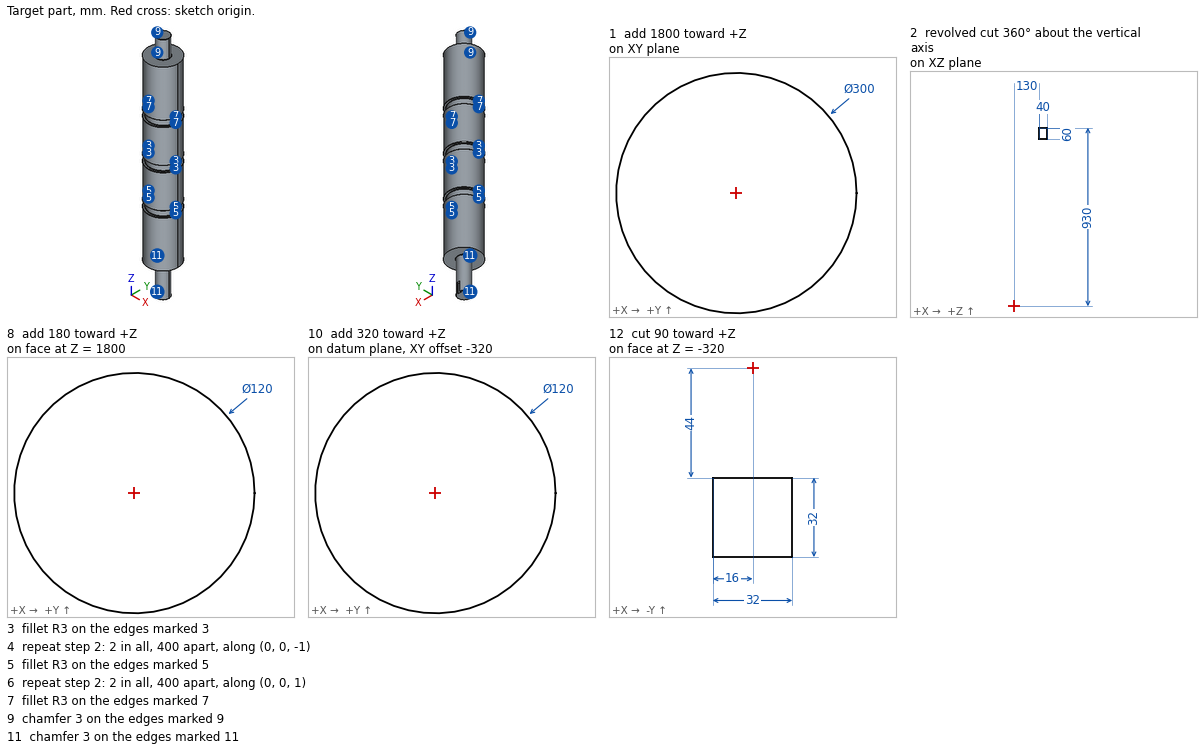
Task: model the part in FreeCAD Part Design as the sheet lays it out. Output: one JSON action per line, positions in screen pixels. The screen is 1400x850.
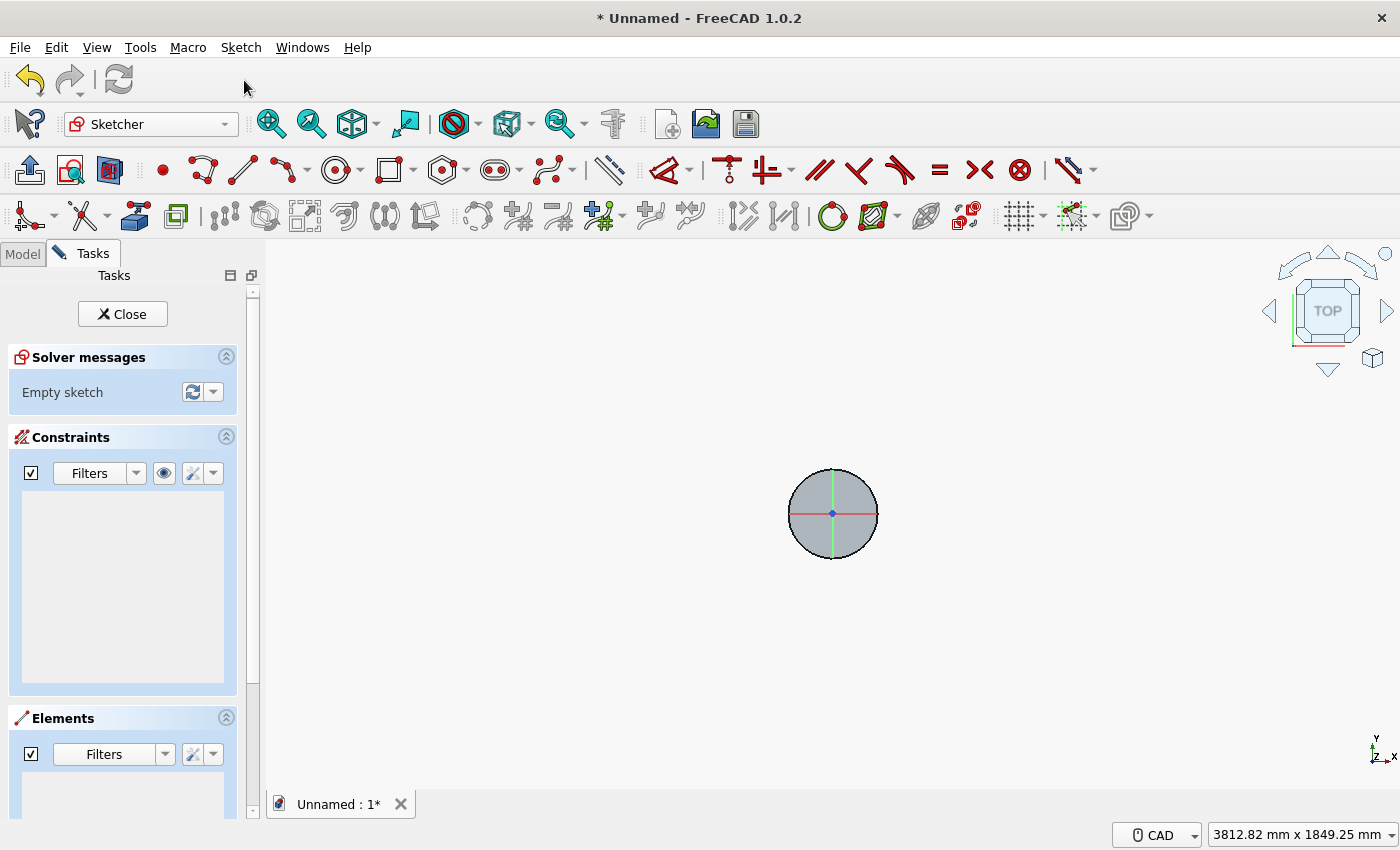
{"action": "scroll", "coordinate": [842, 514], "scroll_direction": "up", "scroll_amount": 11}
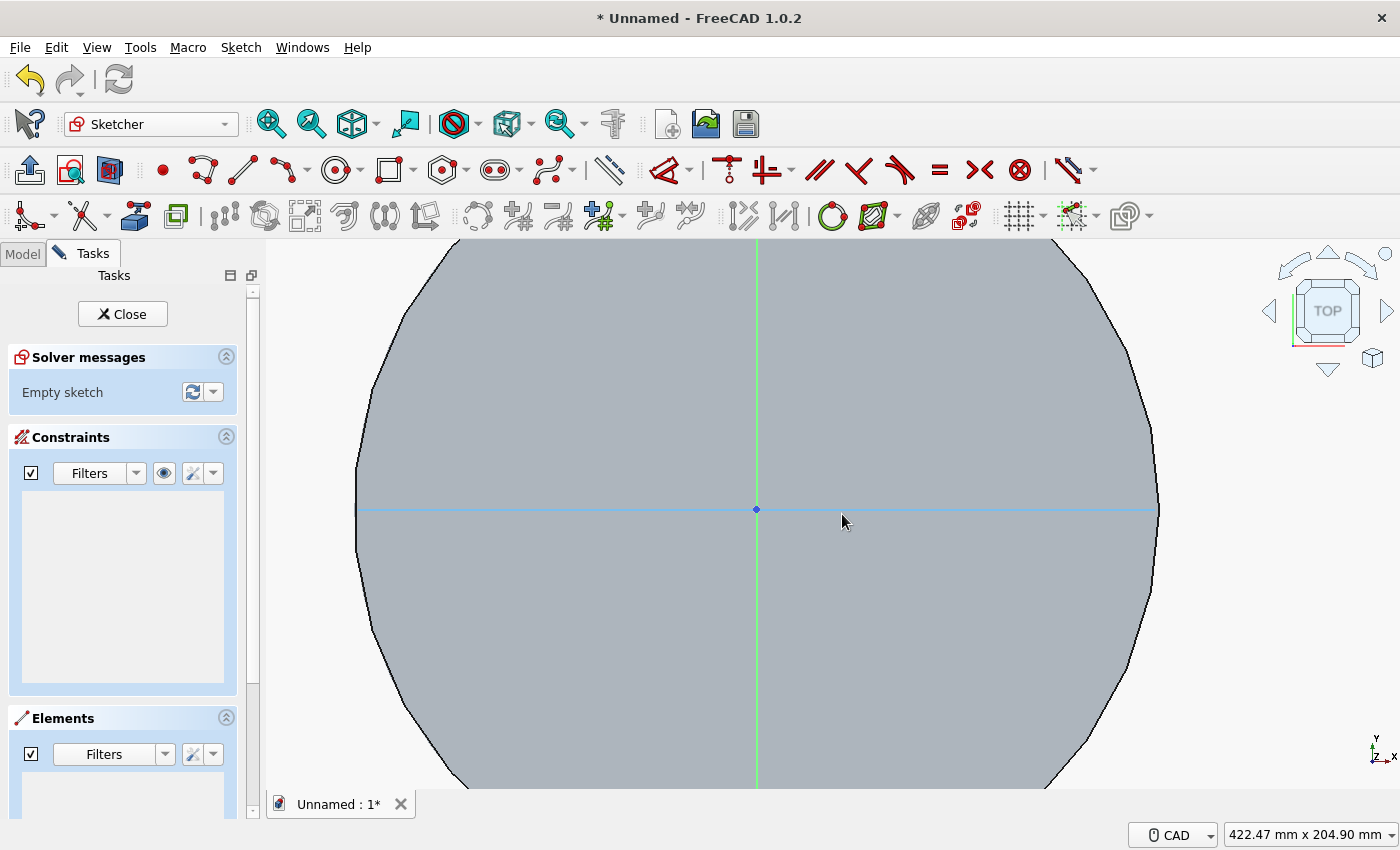
{"action": "left_click", "coordinate": [336, 170]}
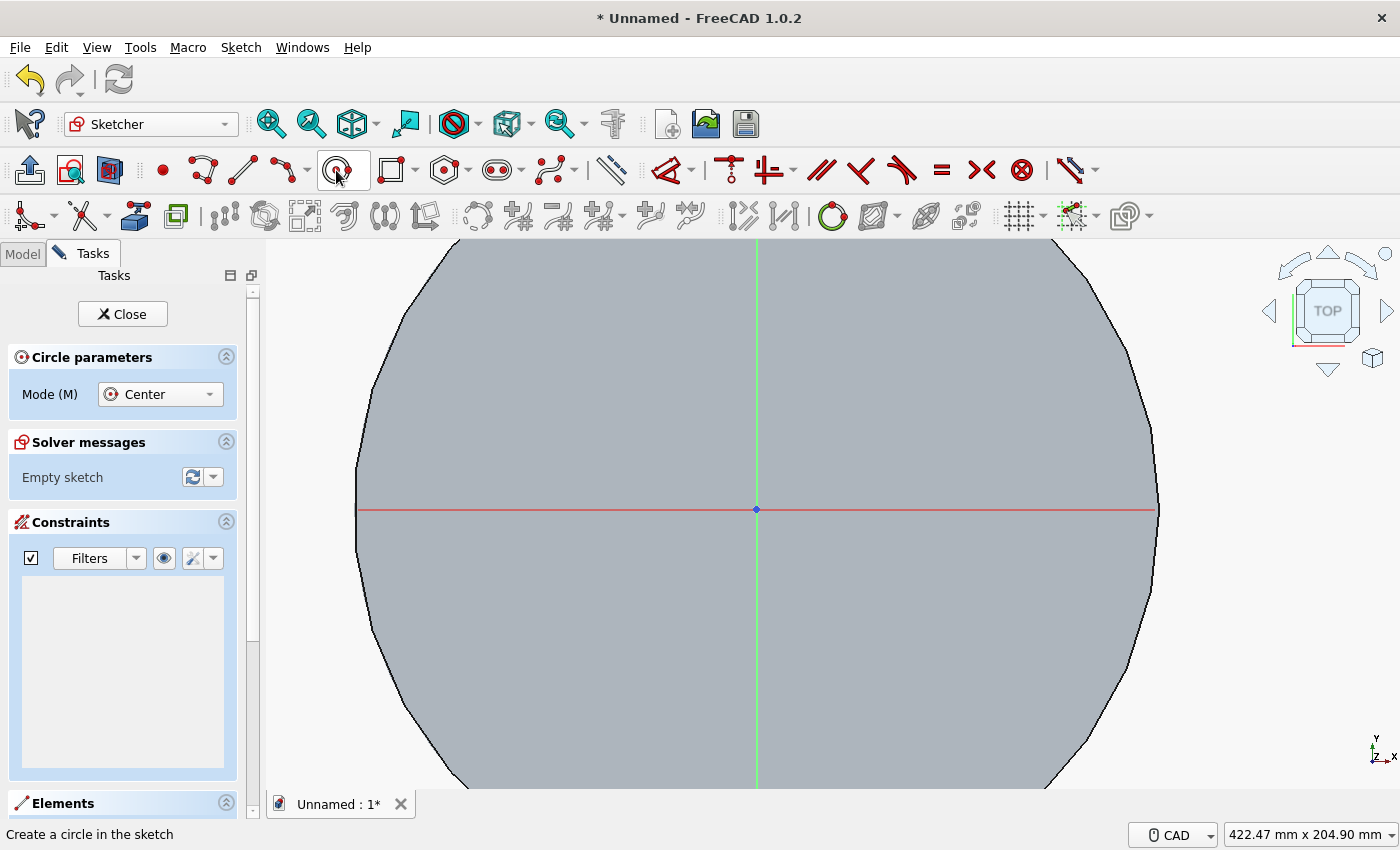
{"action": "left_click", "coordinate": [757, 510]}
{"action": "mouse_move", "coordinate": [870, 396]}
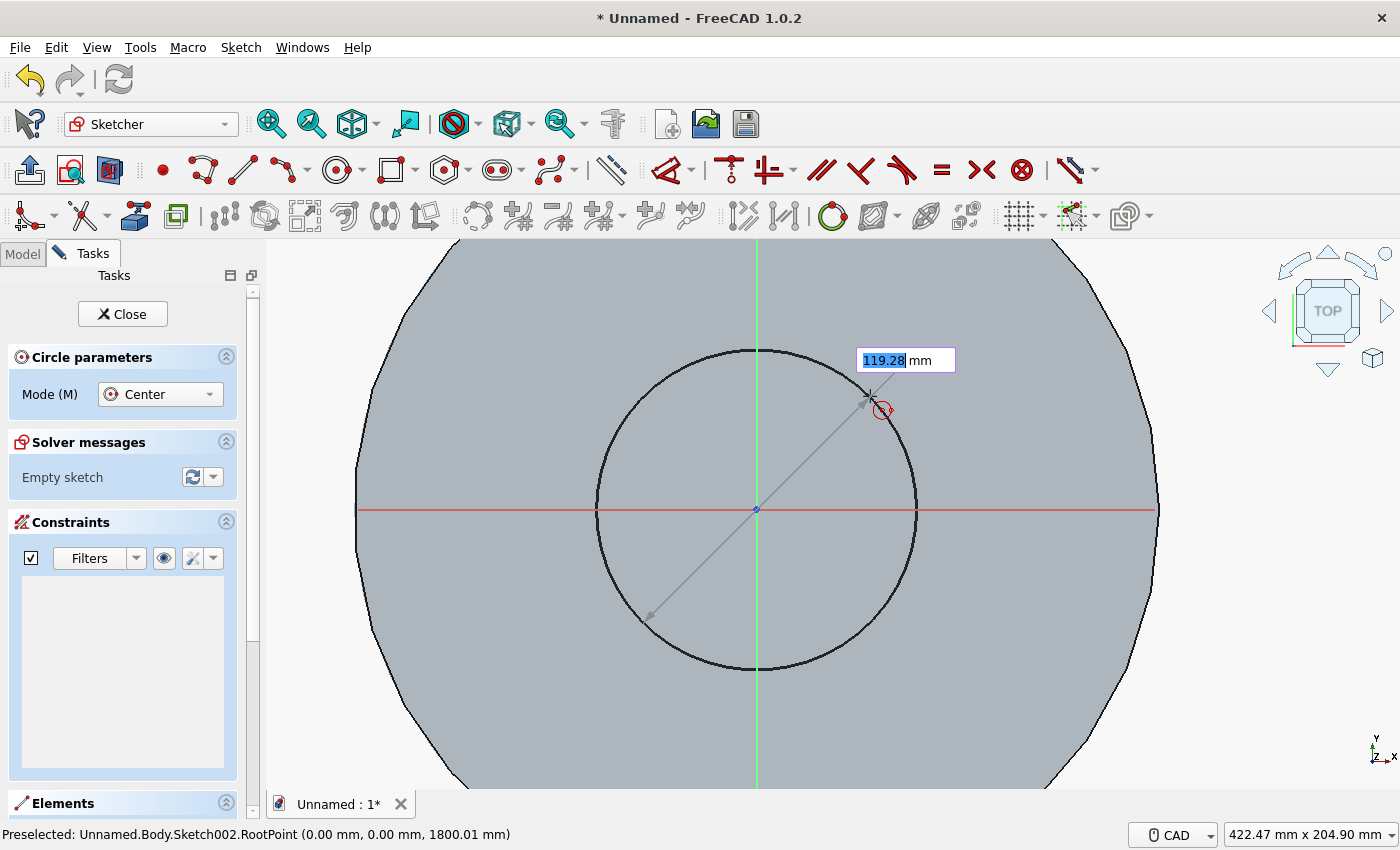
{"action": "type", "text": "120"}
{"action": "key", "text": "Return"}
{"action": "key", "text": "Escape"}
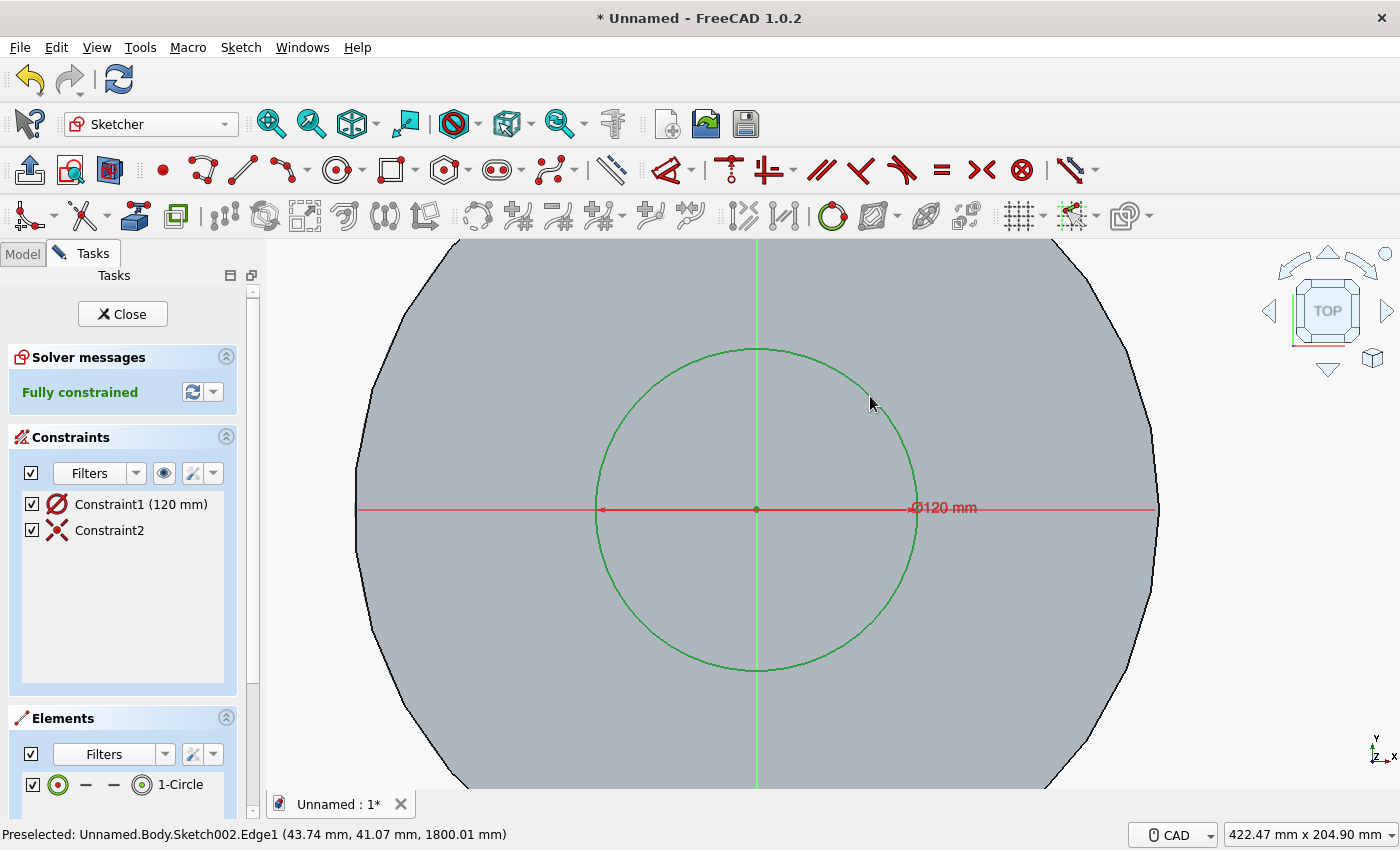
{"action": "left_click", "coordinate": [123, 314]}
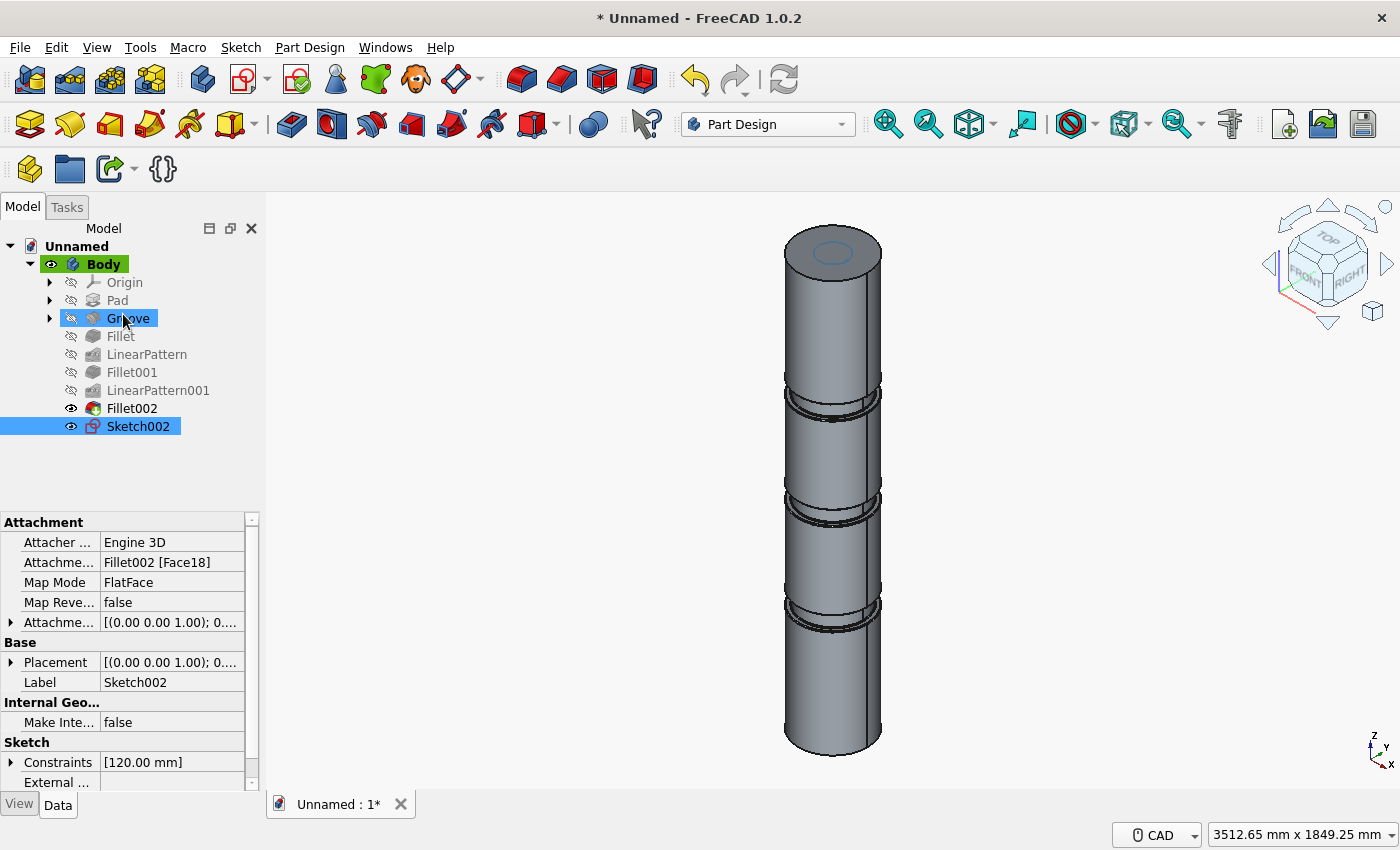
{"action": "left_click", "coordinate": [30, 124]}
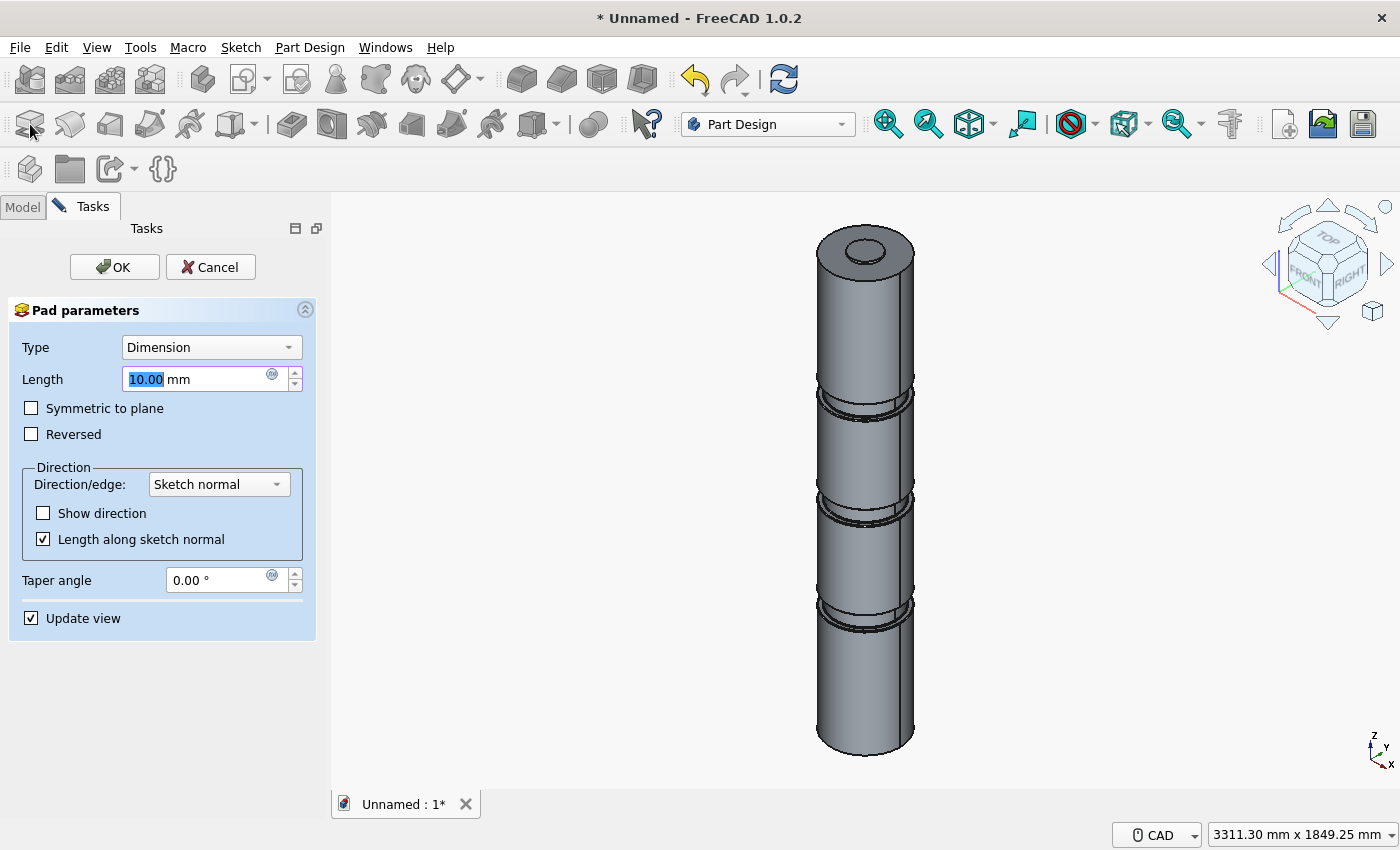
{"action": "type", "text": "180"}
{"action": "key", "text": "Tab"}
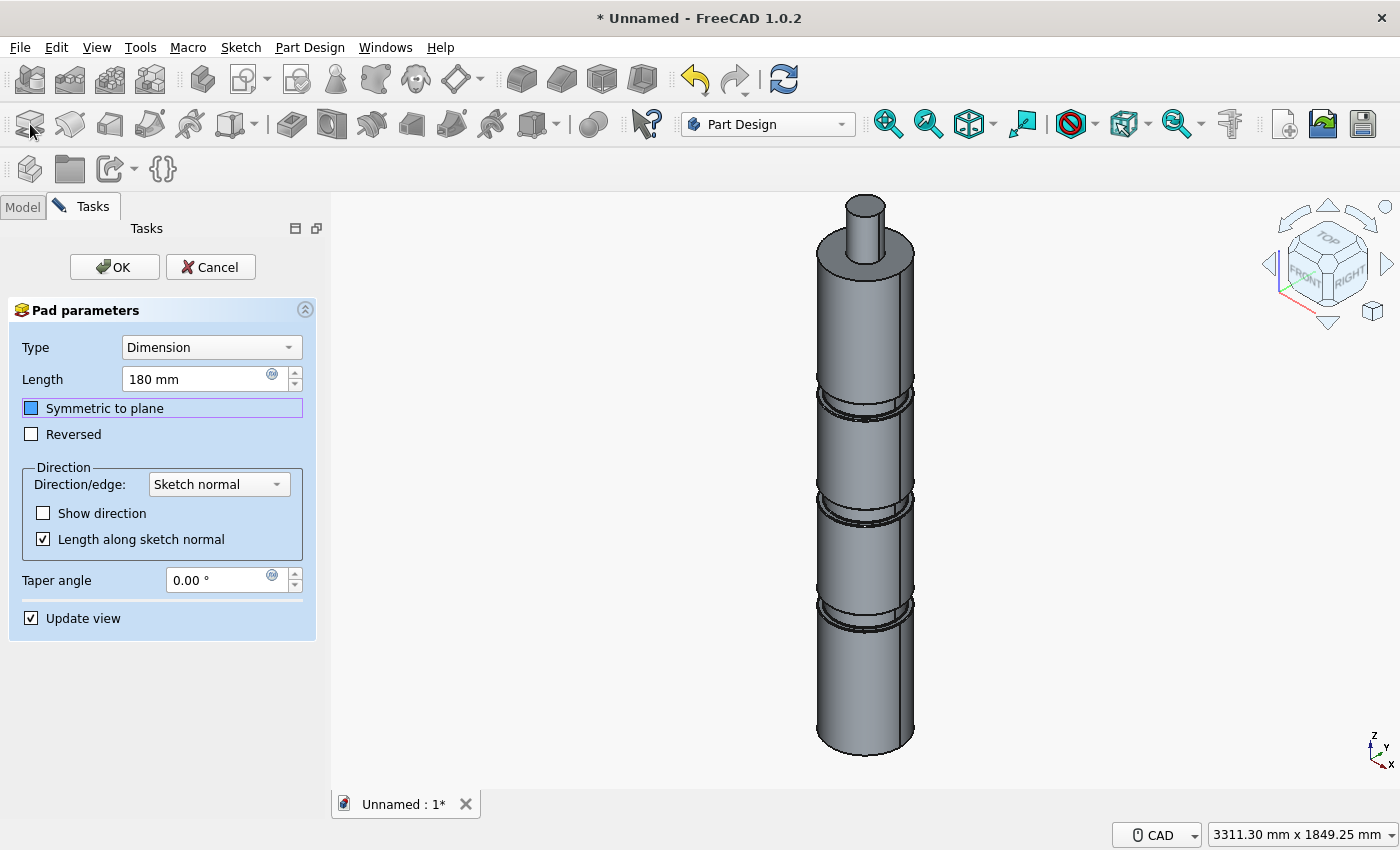
{"action": "left_click", "coordinate": [115, 267]}